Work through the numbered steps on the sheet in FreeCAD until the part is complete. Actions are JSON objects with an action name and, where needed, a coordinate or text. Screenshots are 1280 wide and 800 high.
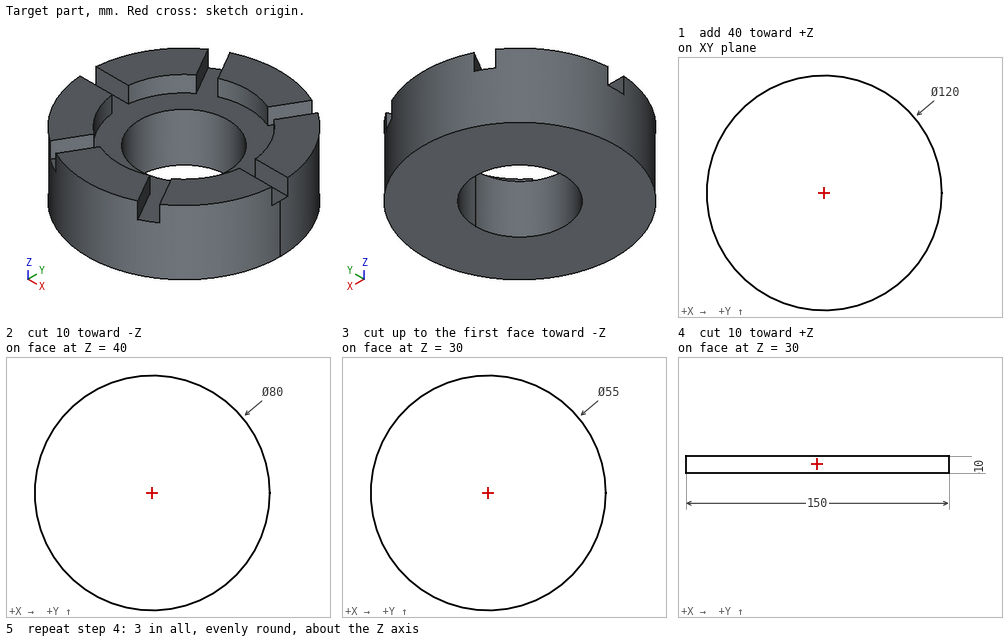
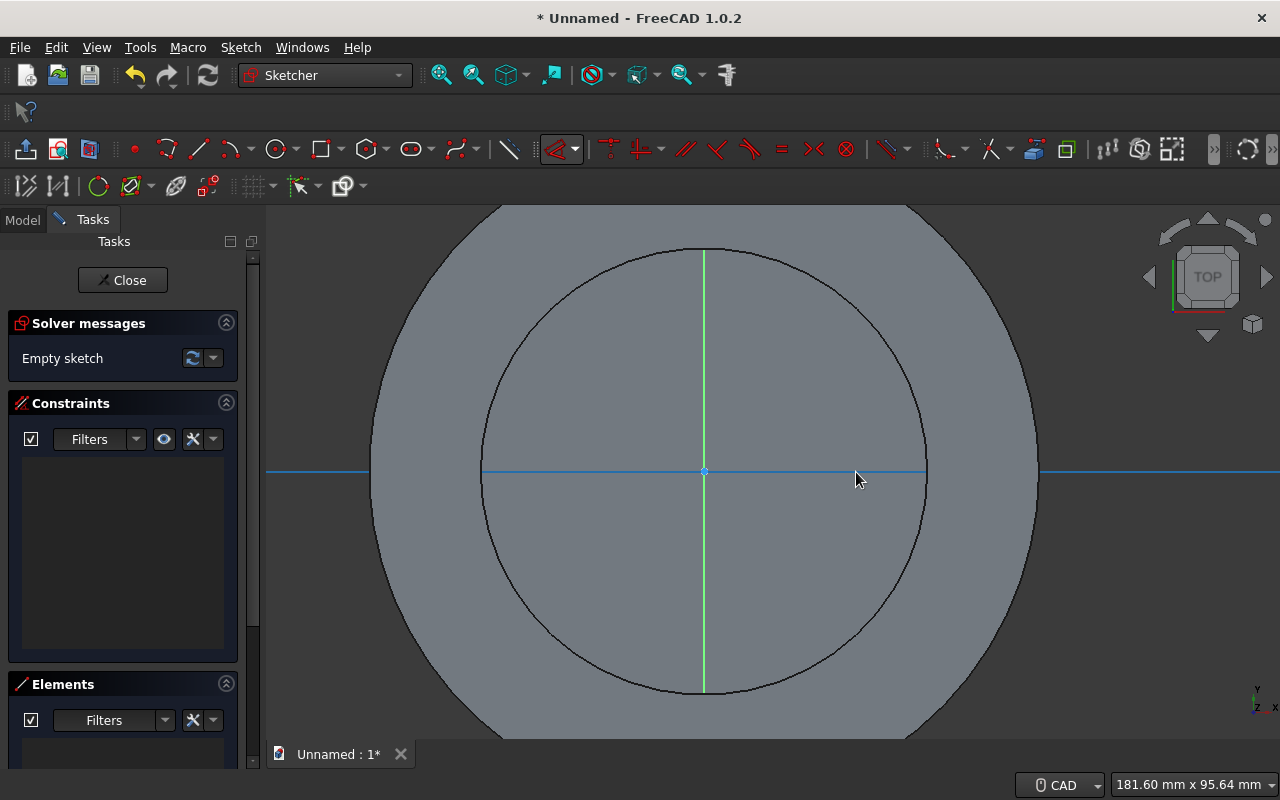
{"action": "key", "text": "g c"}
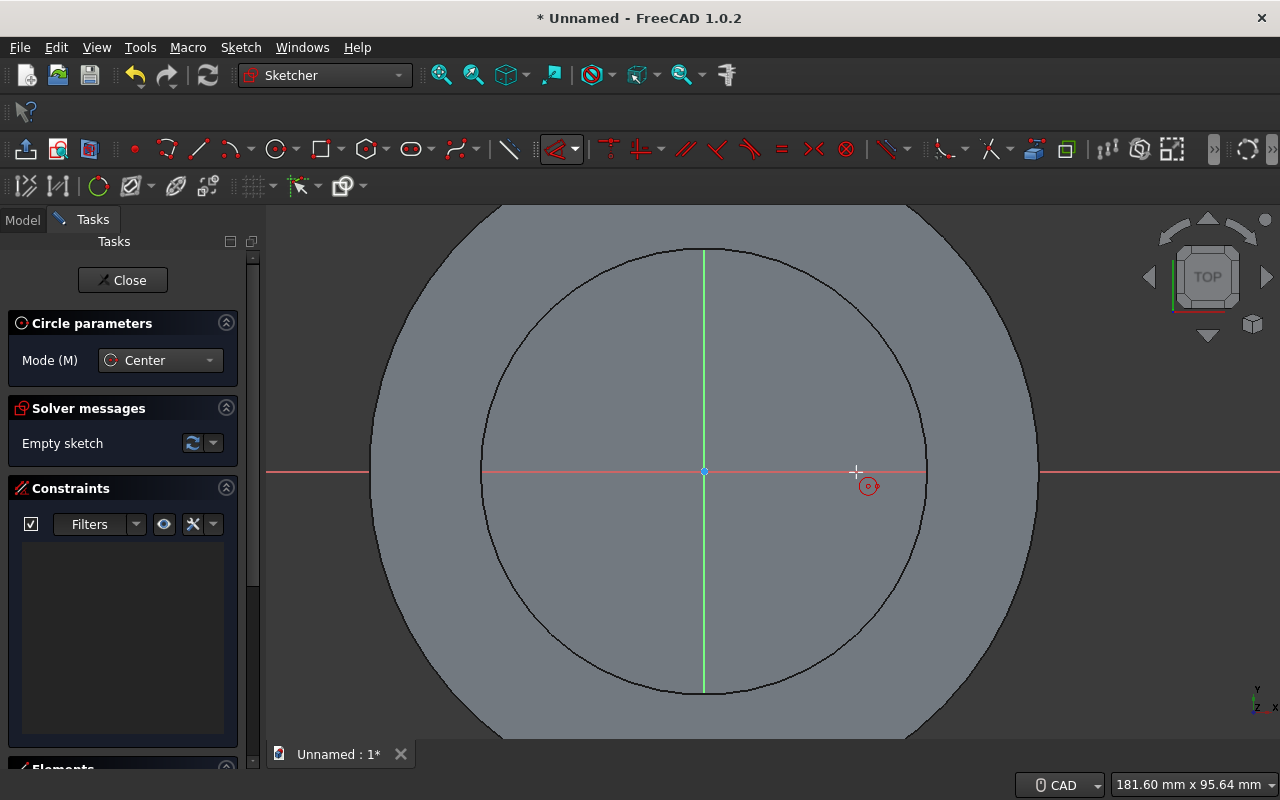
{"action": "left_click", "coordinate": [704, 472]}
{"action": "left_click", "coordinate": [813, 363]}
{"action": "key", "text": "Escape"}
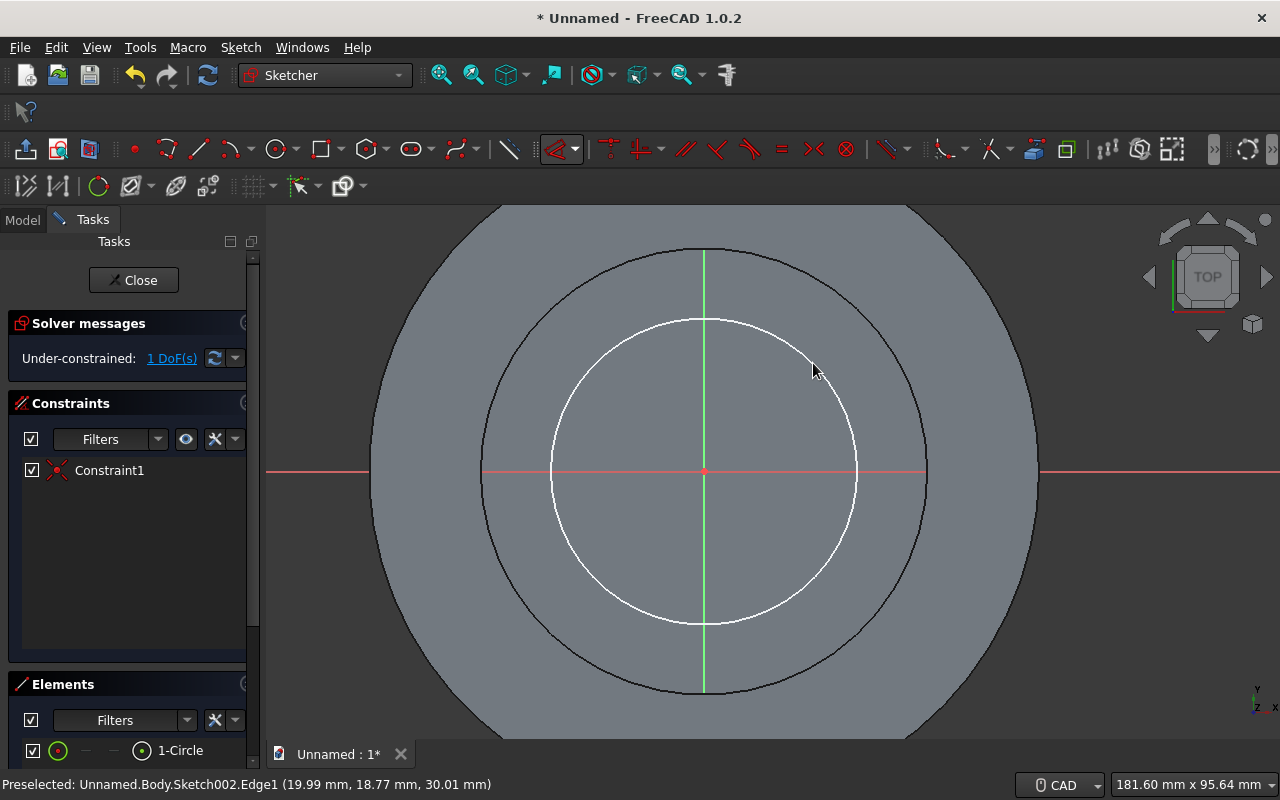
{"action": "left_click", "coordinate": [556, 150]}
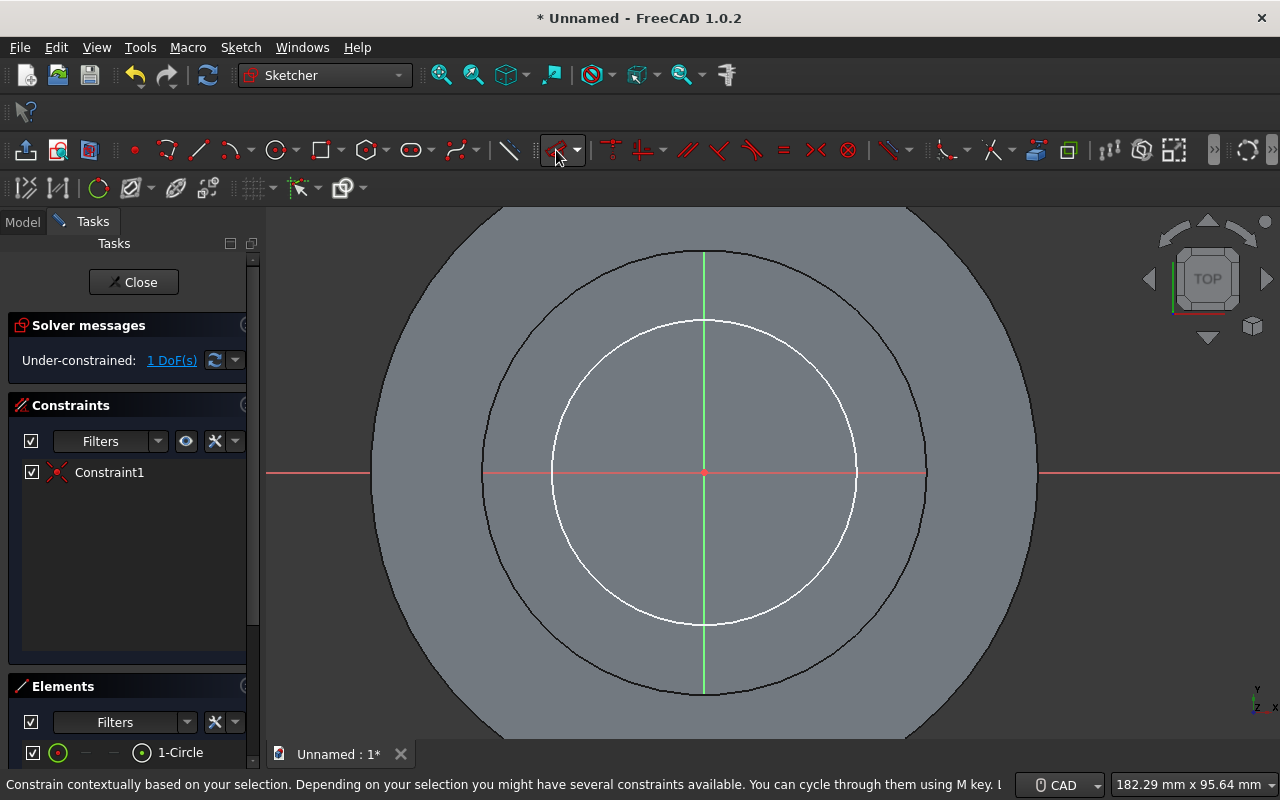
{"action": "left_click", "coordinate": [812, 364]}
{"action": "left_click", "coordinate": [835, 341]}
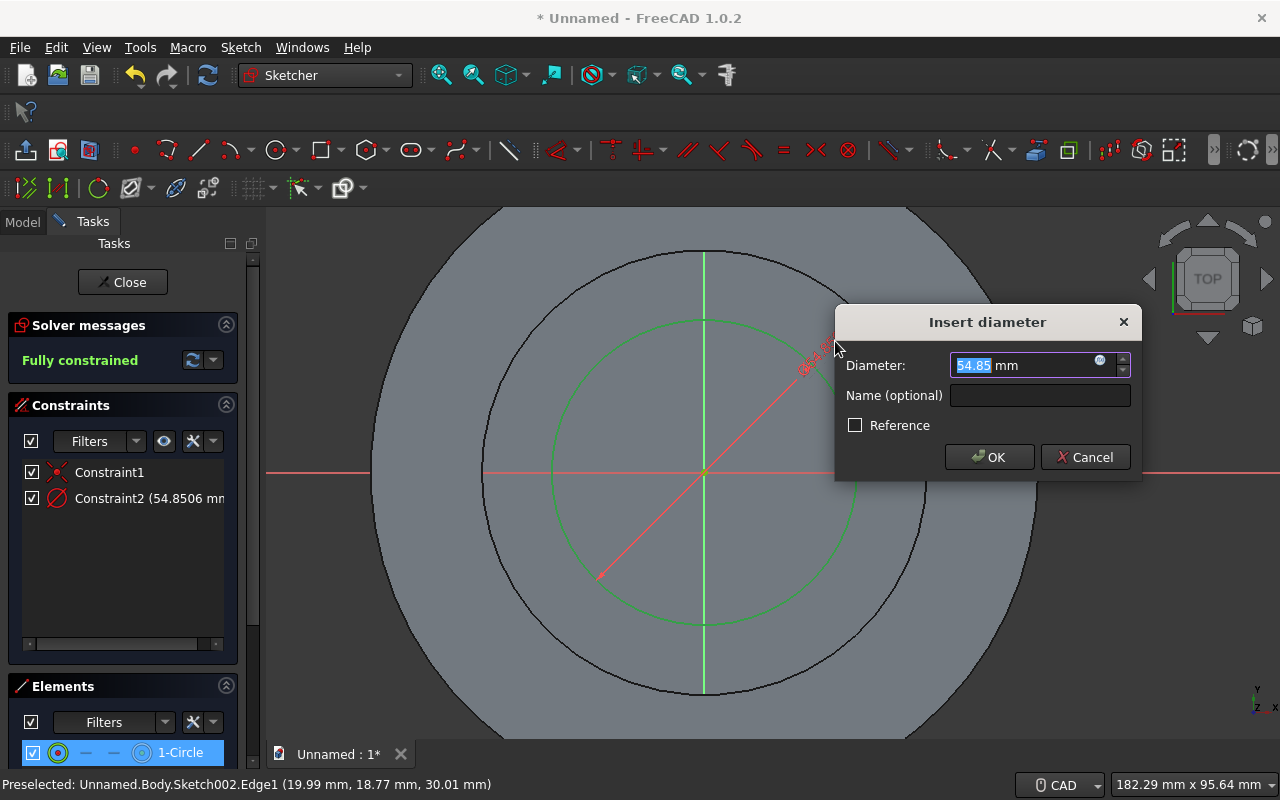
{"action": "type", "text": "55"}
{"action": "key", "text": "Return"}
{"action": "key", "text": "Escape"}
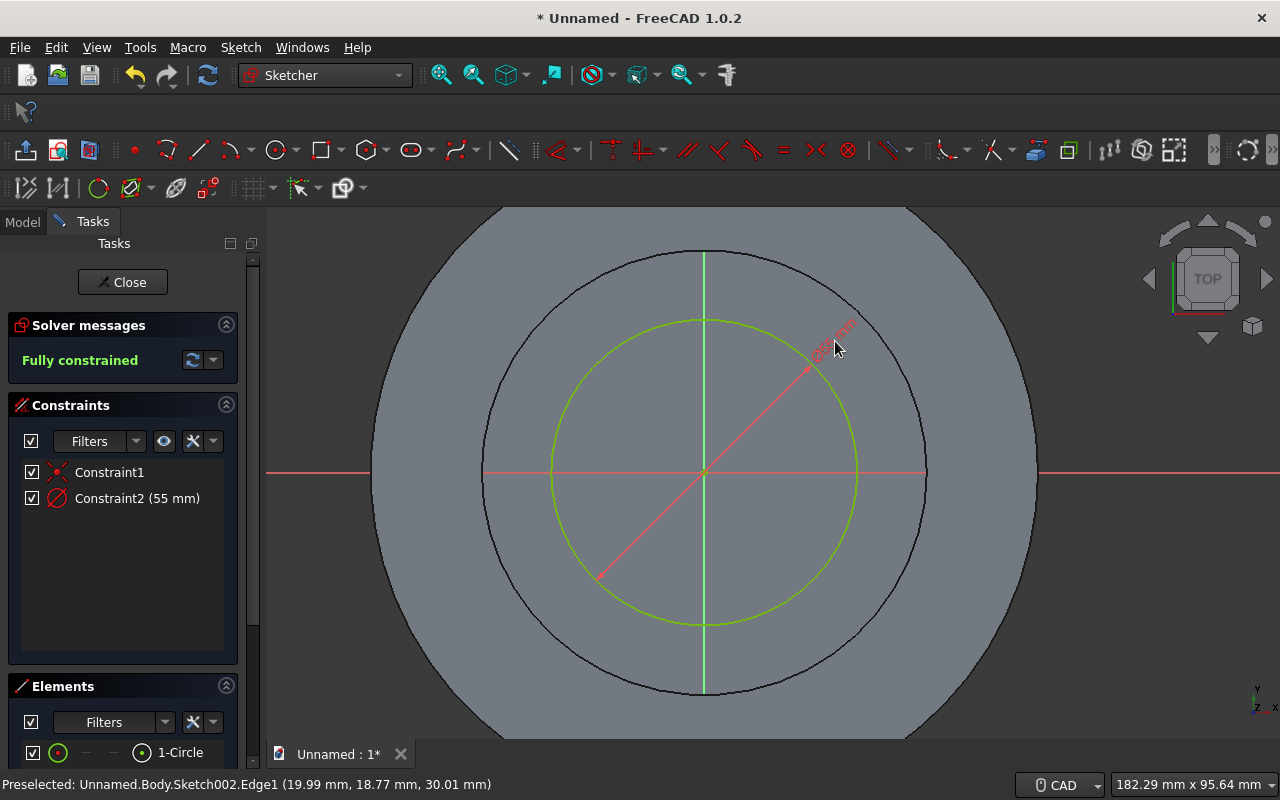
{"action": "left_click", "coordinate": [123, 282]}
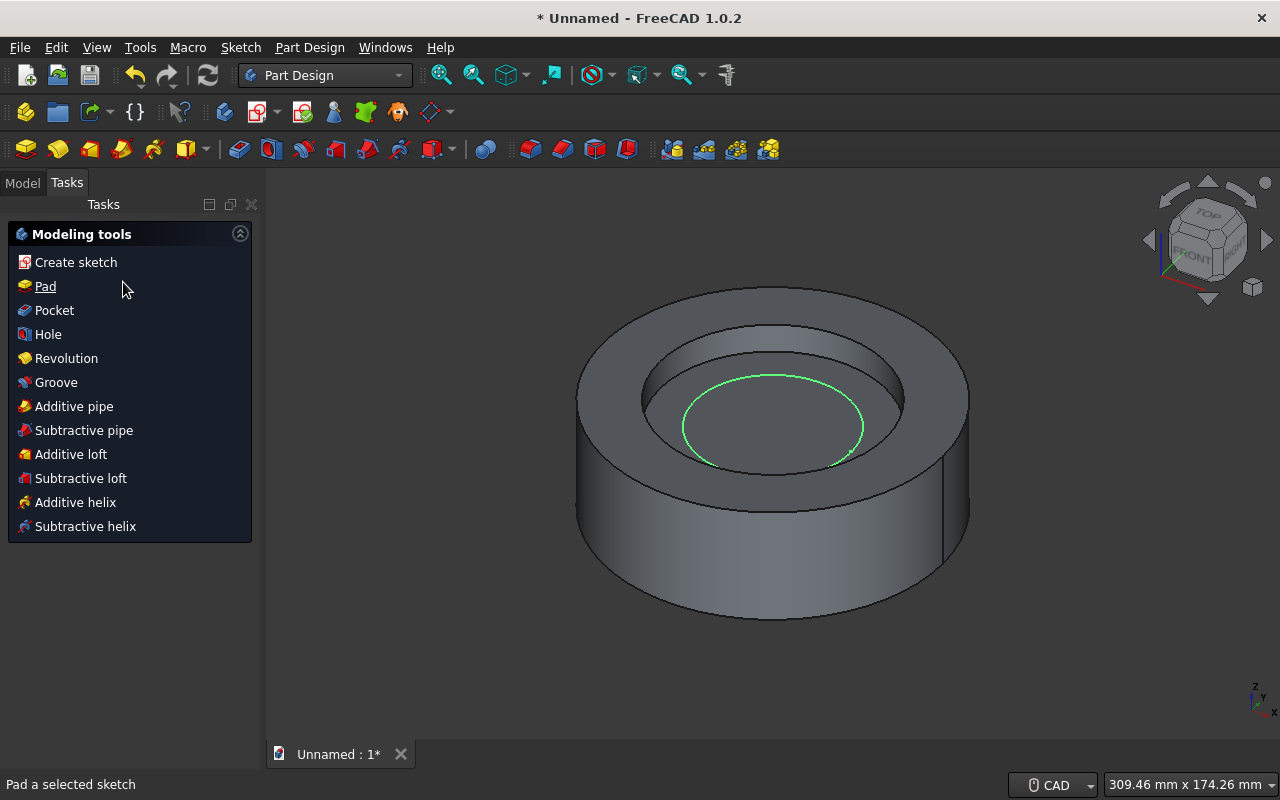
{"action": "left_click", "coordinate": [240, 150]}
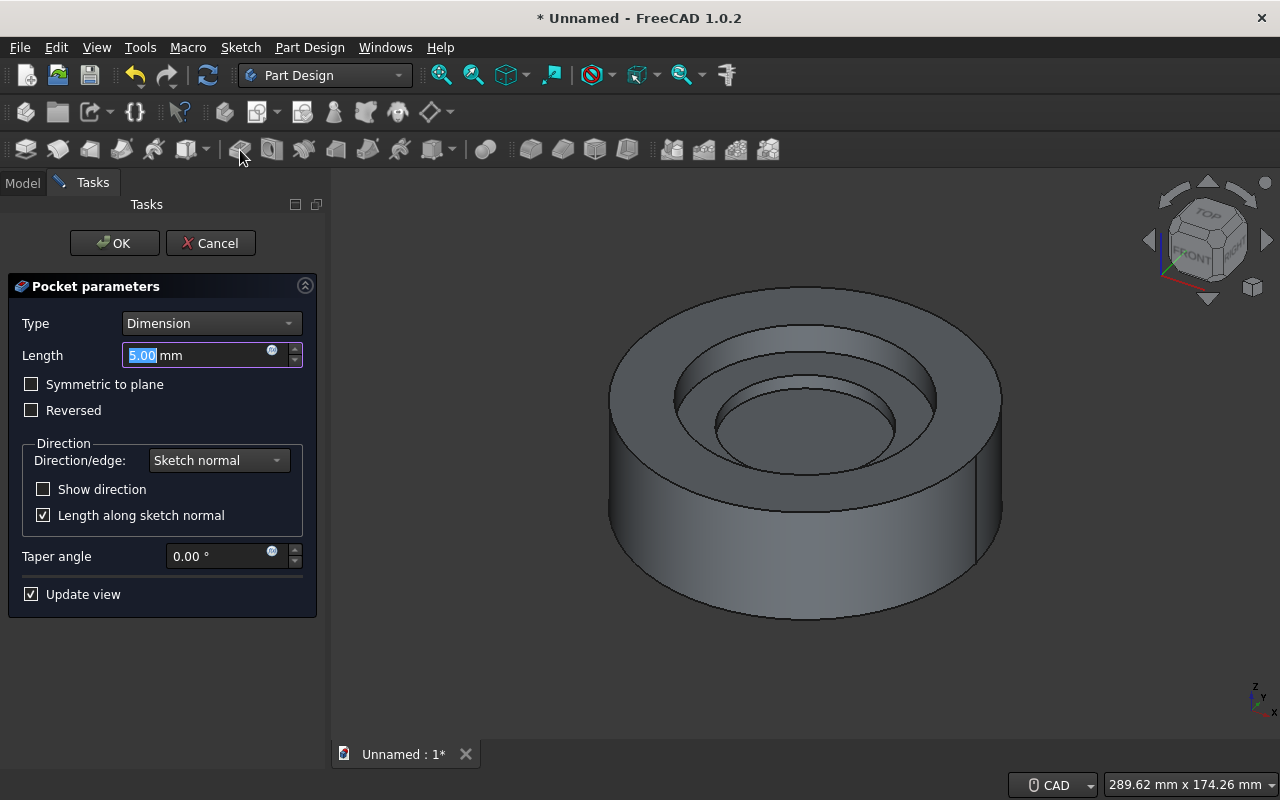
{"action": "left_click", "coordinate": [212, 324]}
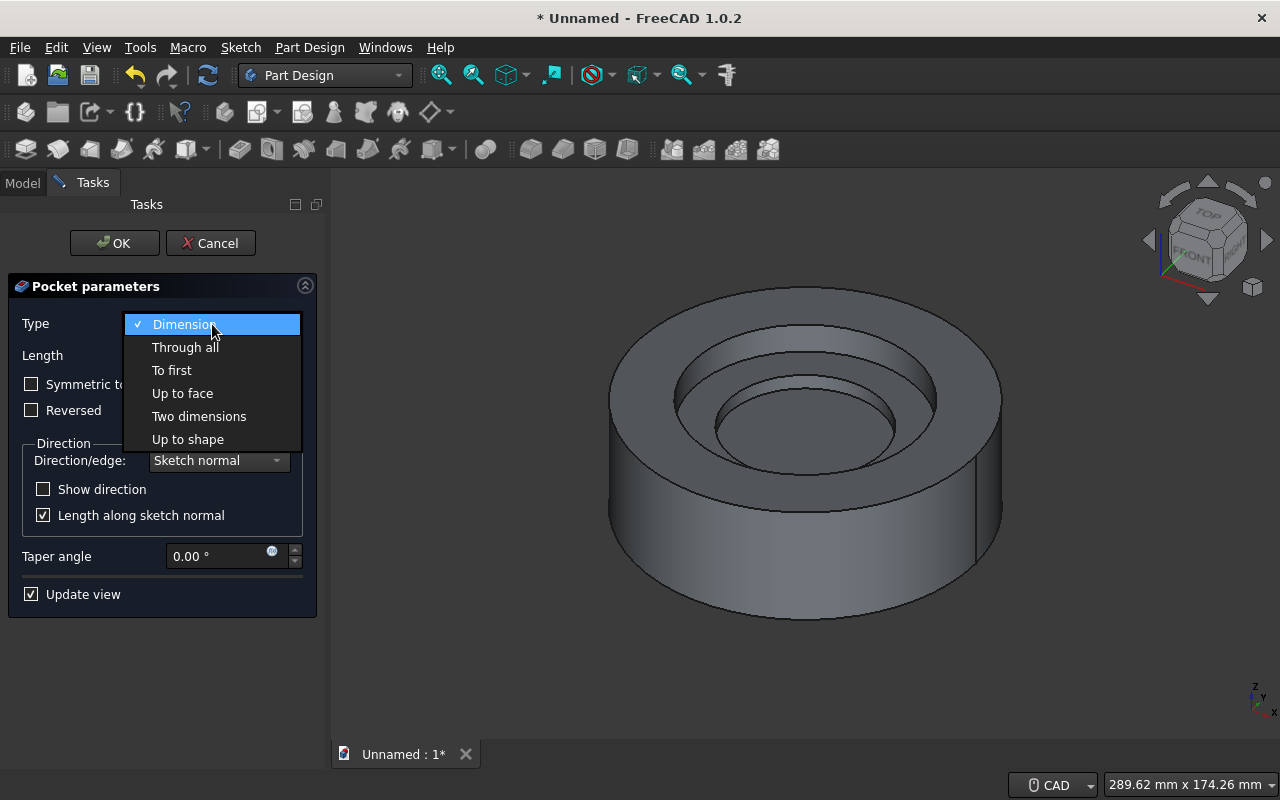
{"action": "left_click", "coordinate": [212, 370]}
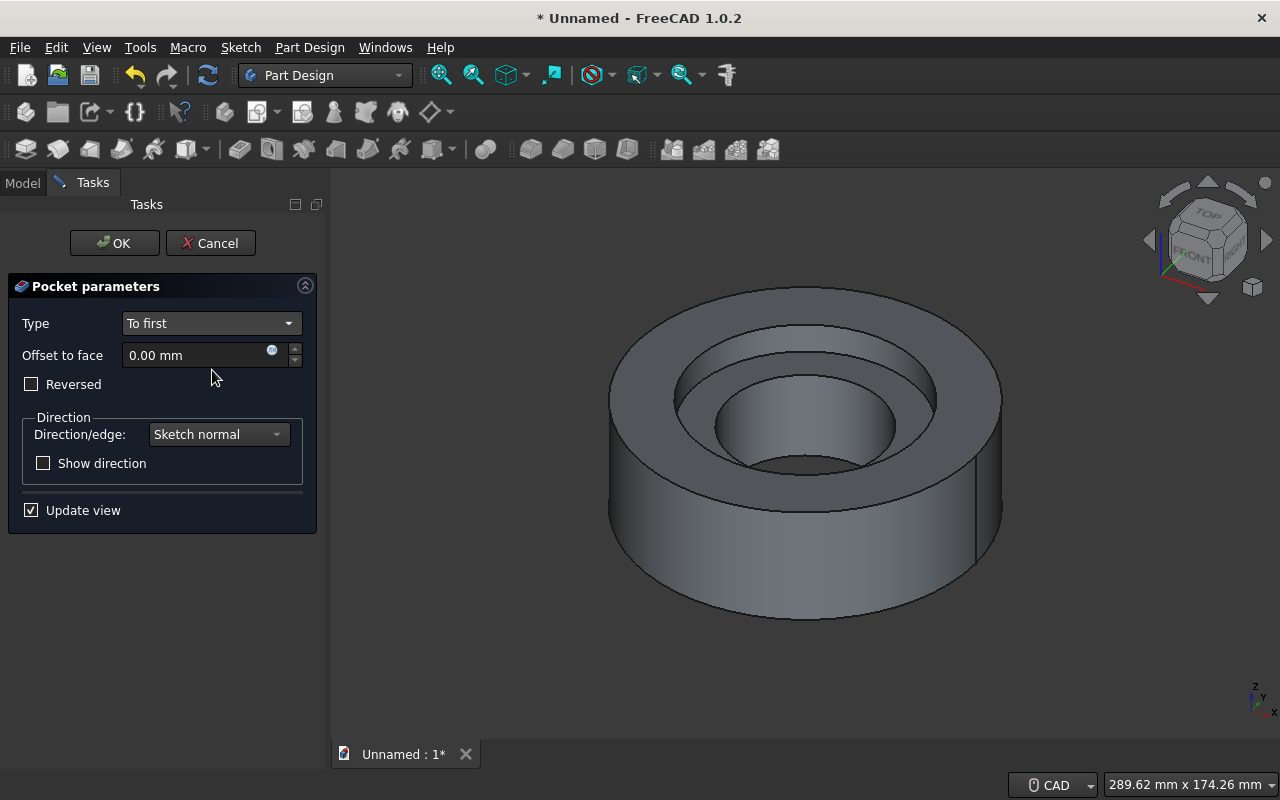
{"action": "left_click", "coordinate": [115, 243]}